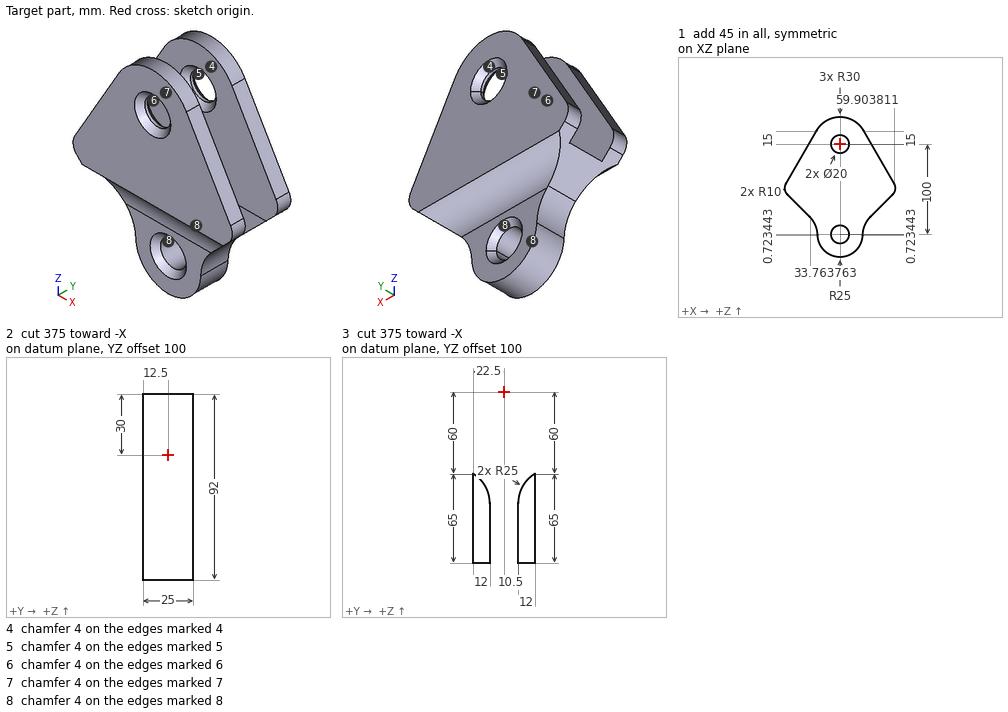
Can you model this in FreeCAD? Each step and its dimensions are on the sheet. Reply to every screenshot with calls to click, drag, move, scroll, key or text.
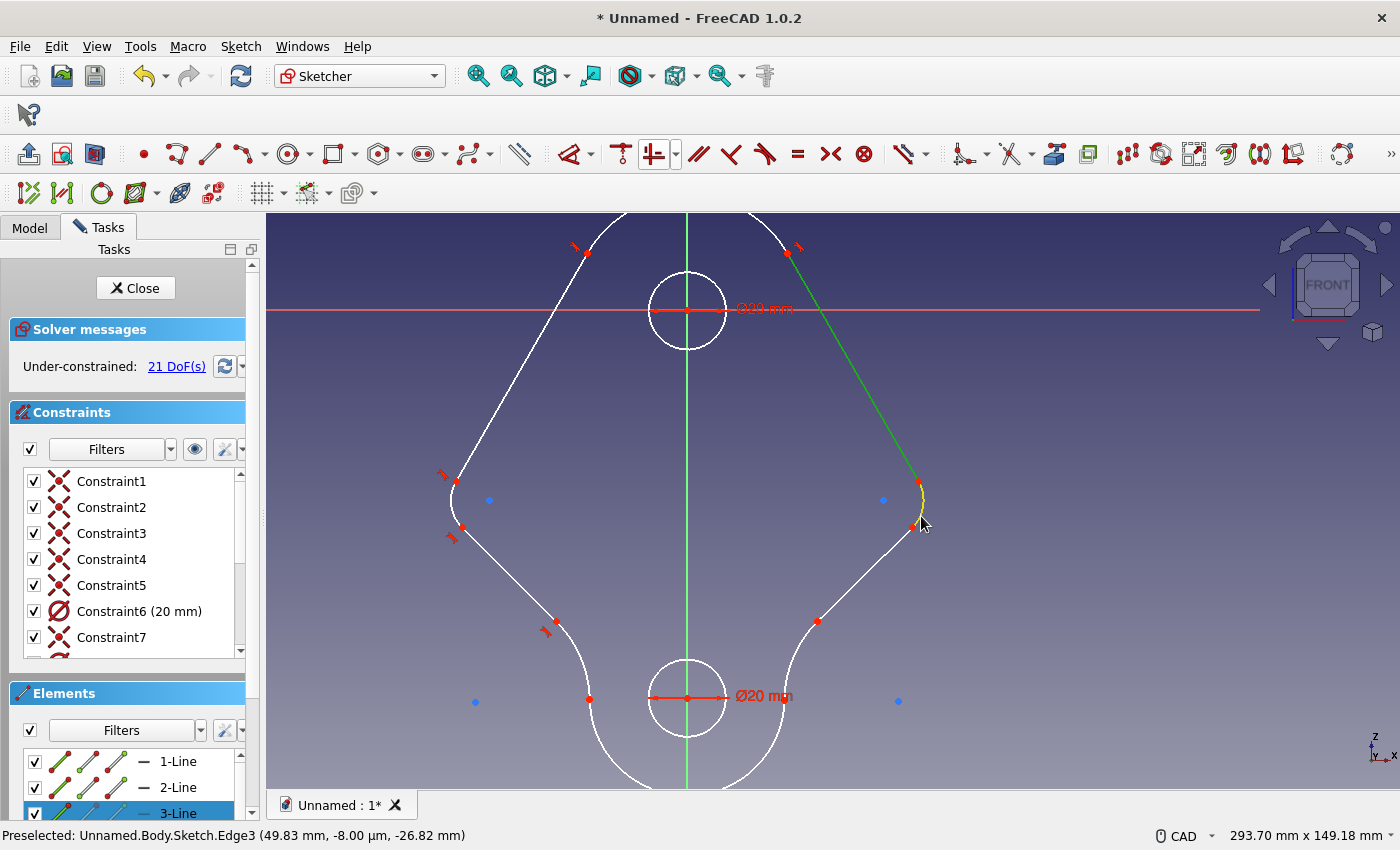
click(921, 515)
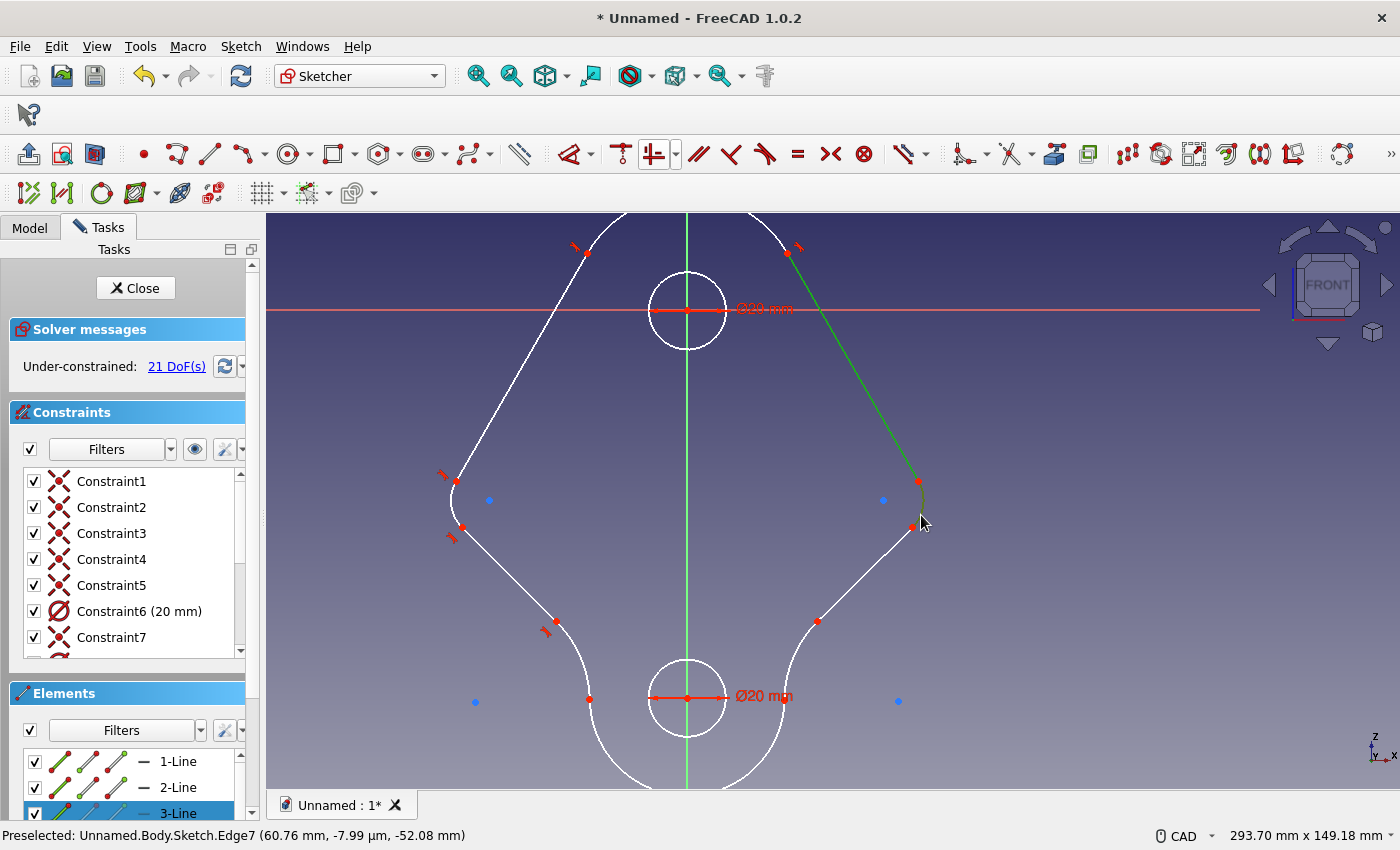
click(765, 154)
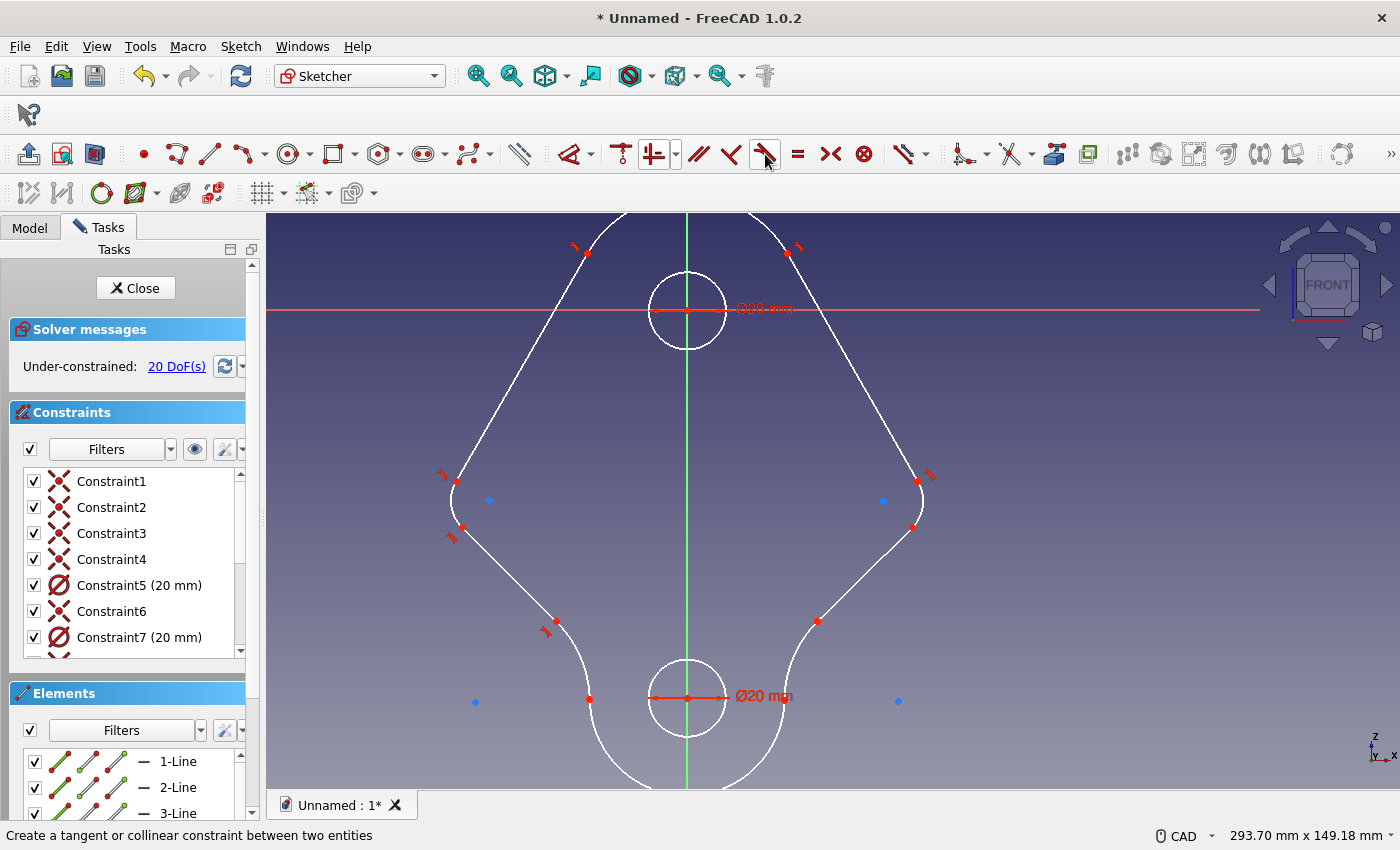
click(884, 556)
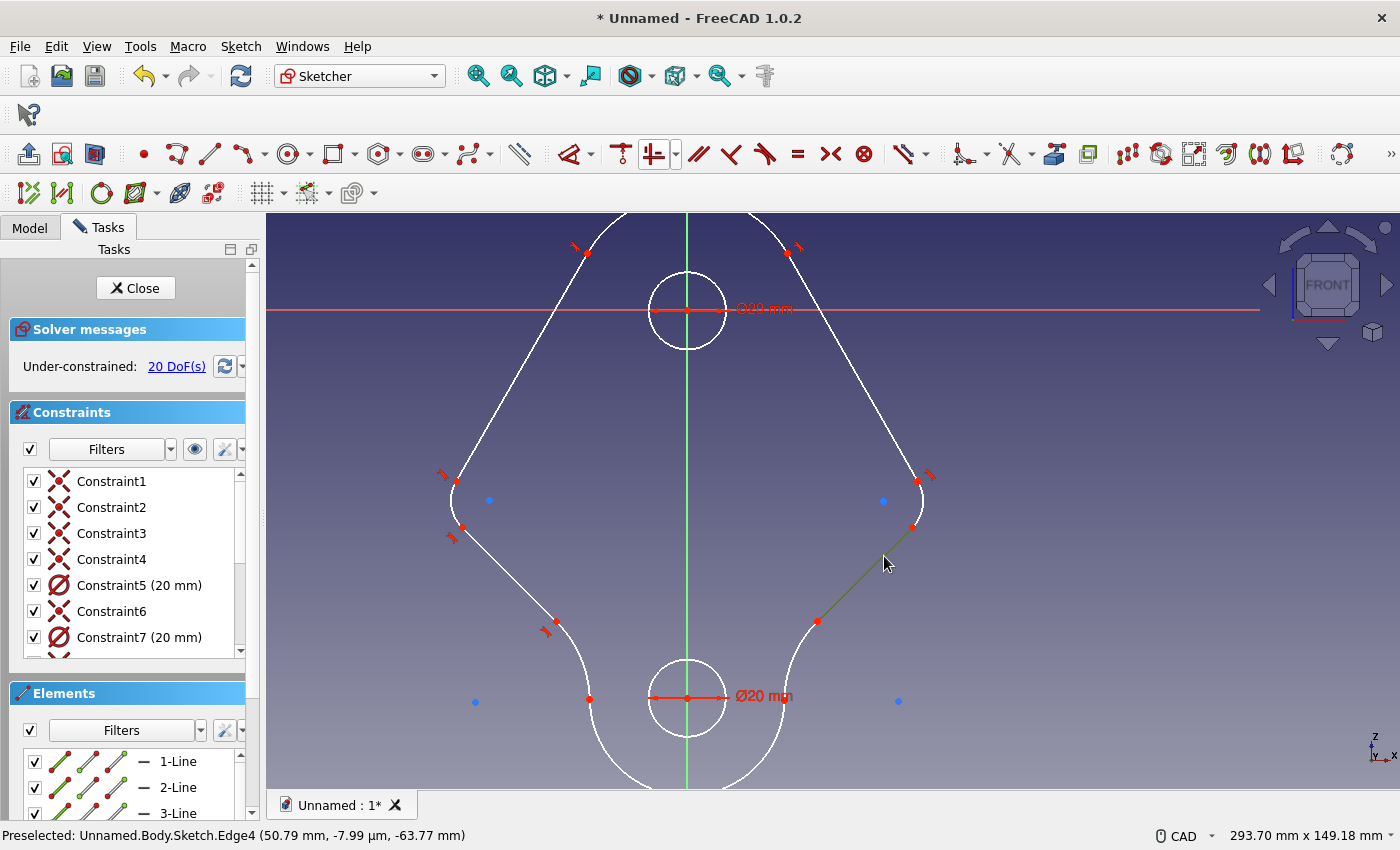
click(921, 515)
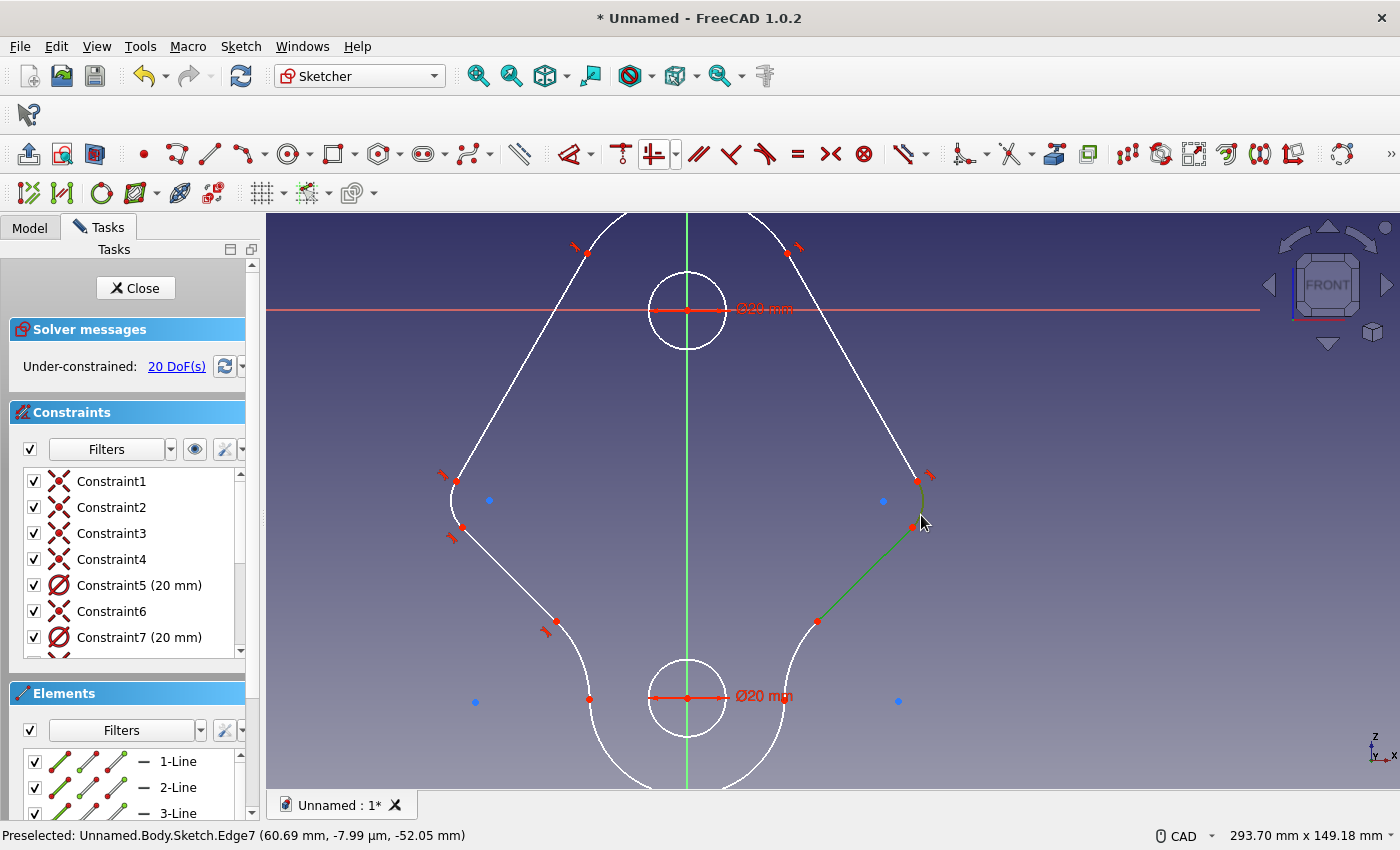
click(765, 154)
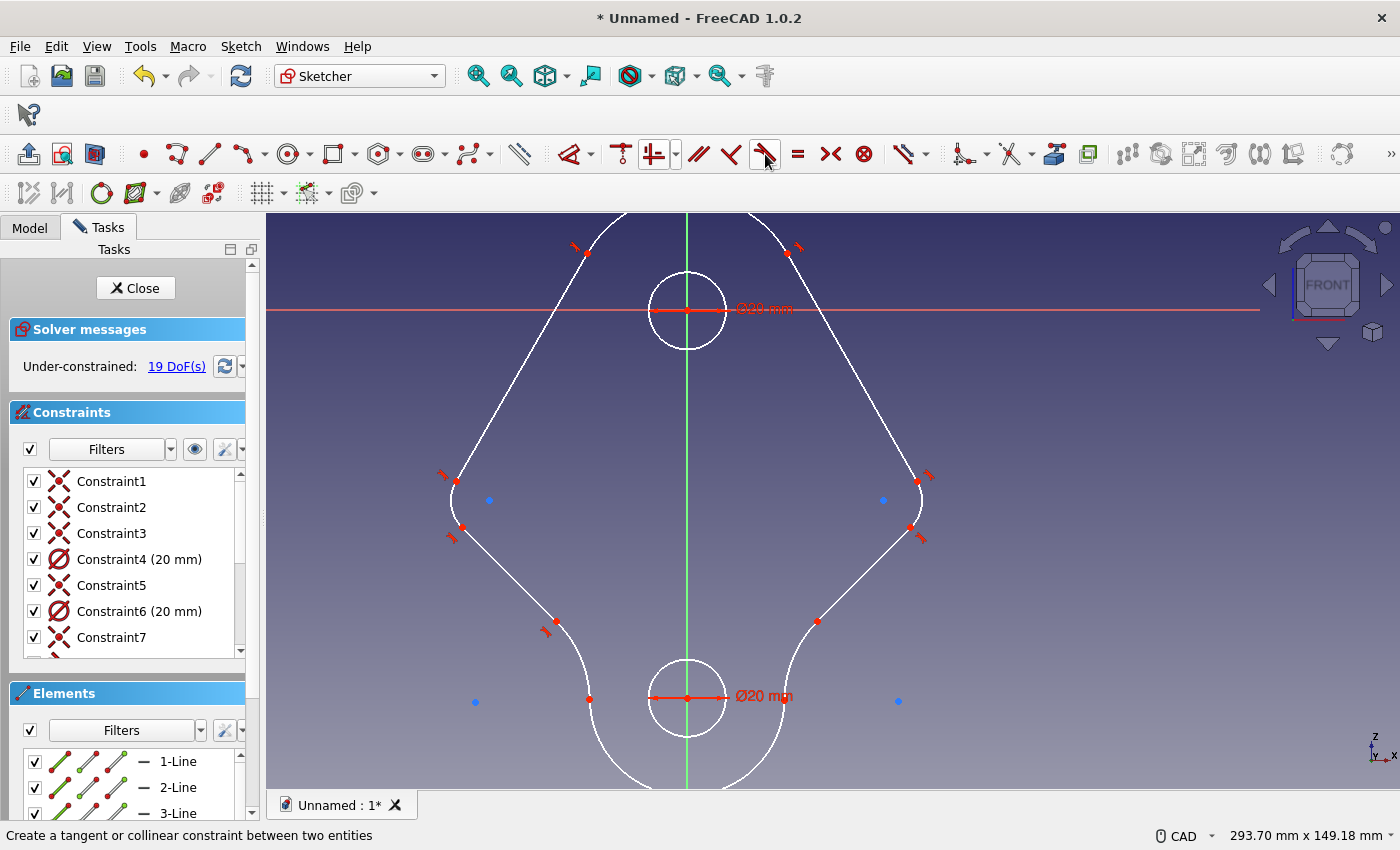
click(883, 556)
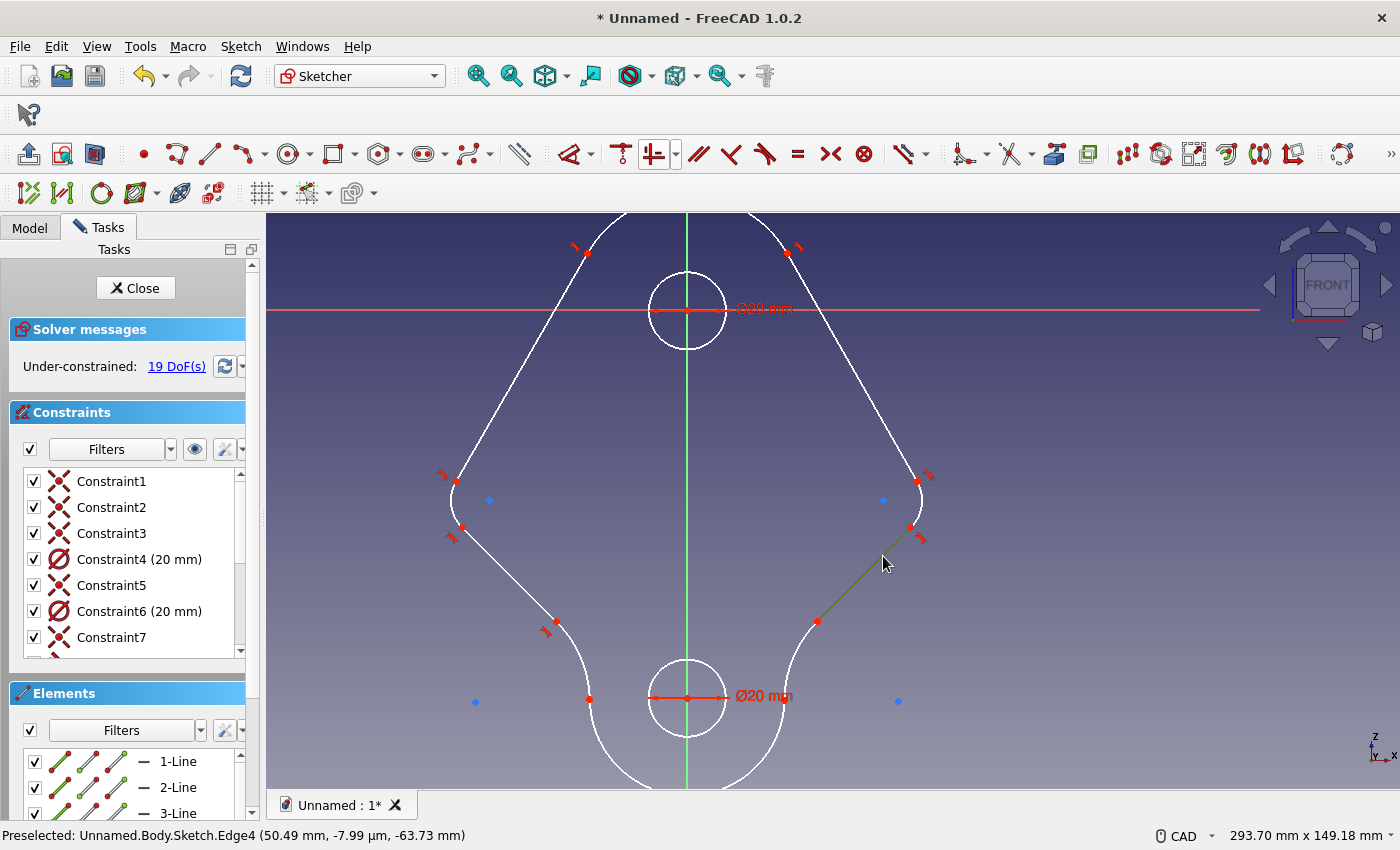
click(801, 642)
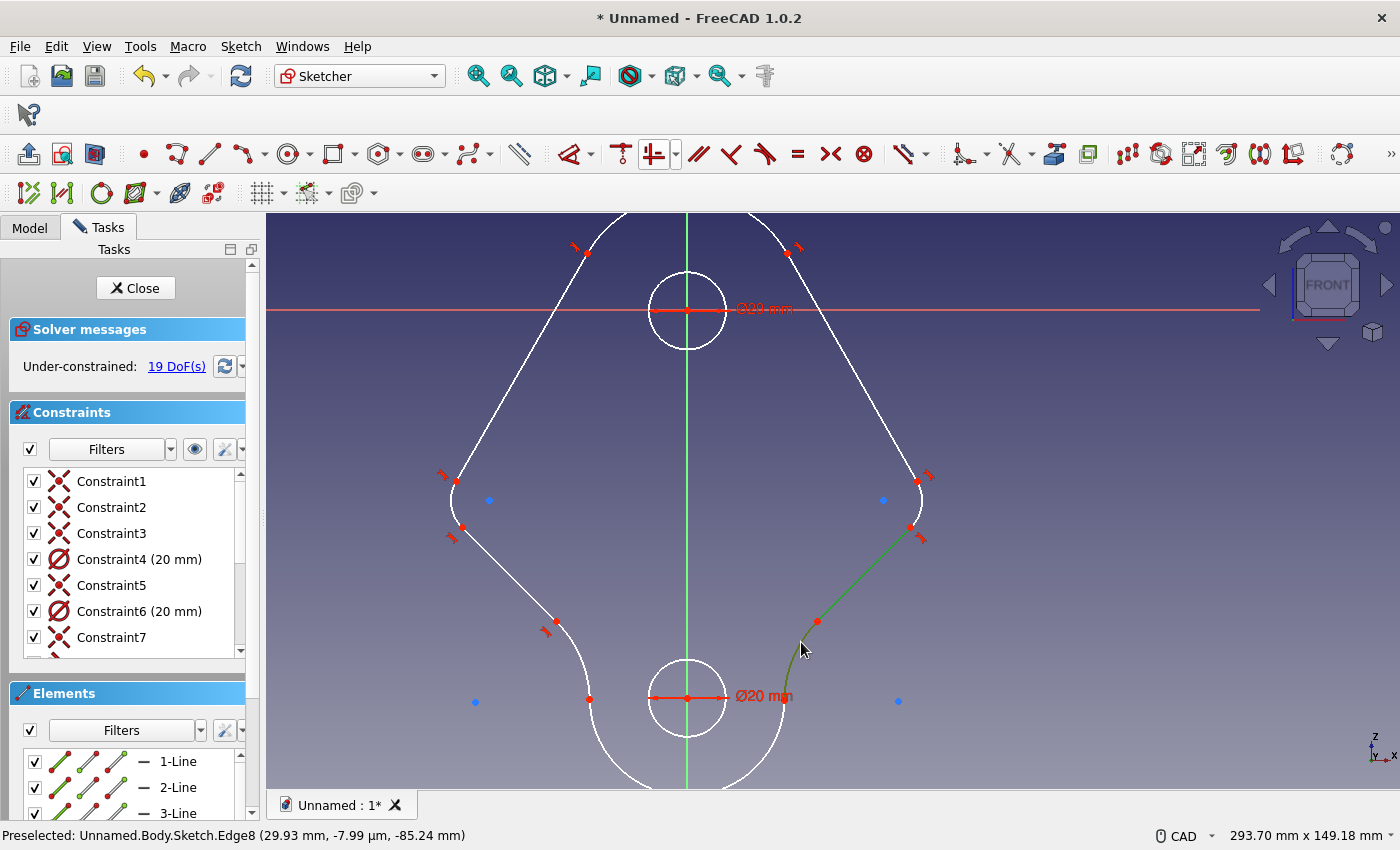
click(765, 154)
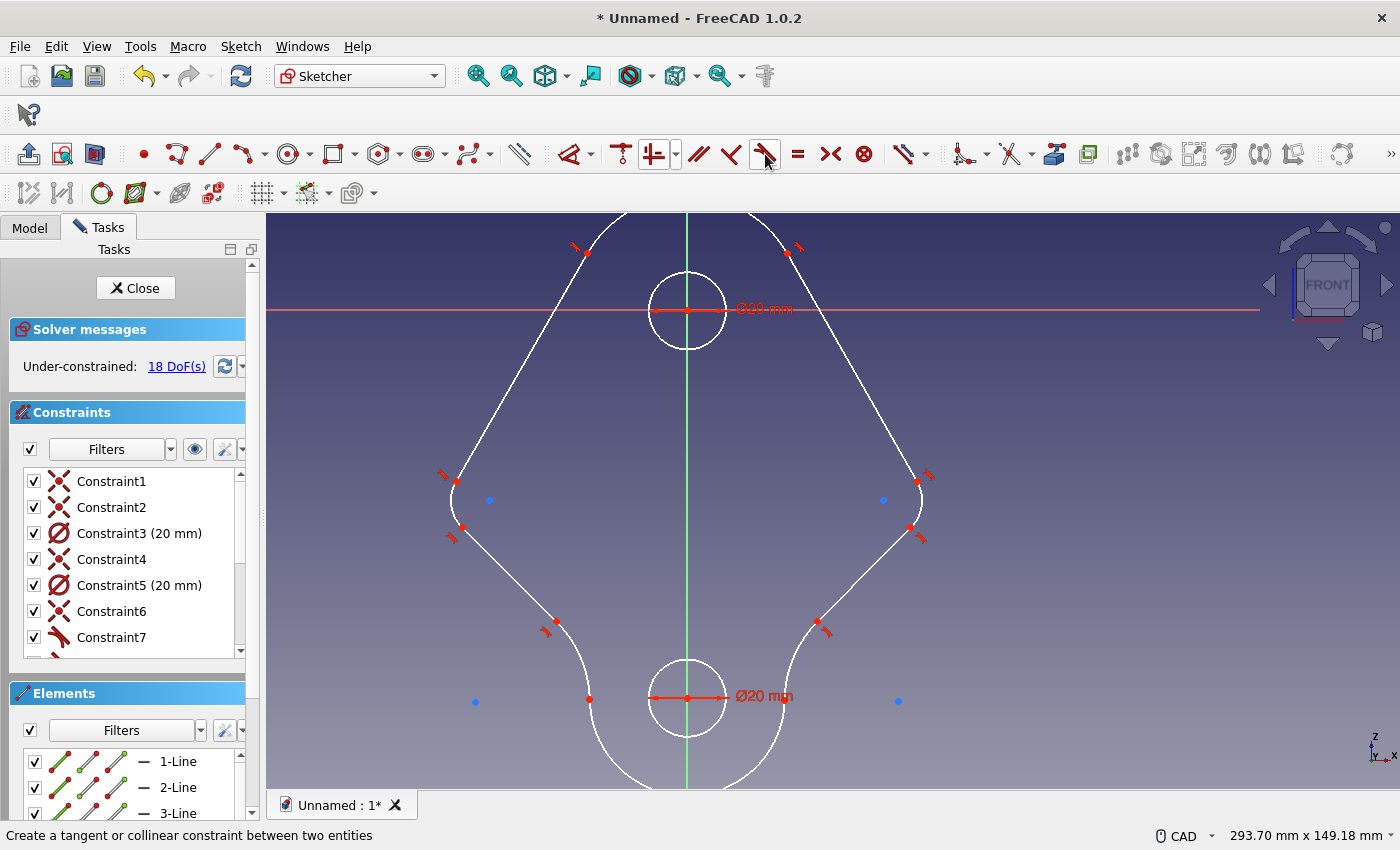
click(801, 642)